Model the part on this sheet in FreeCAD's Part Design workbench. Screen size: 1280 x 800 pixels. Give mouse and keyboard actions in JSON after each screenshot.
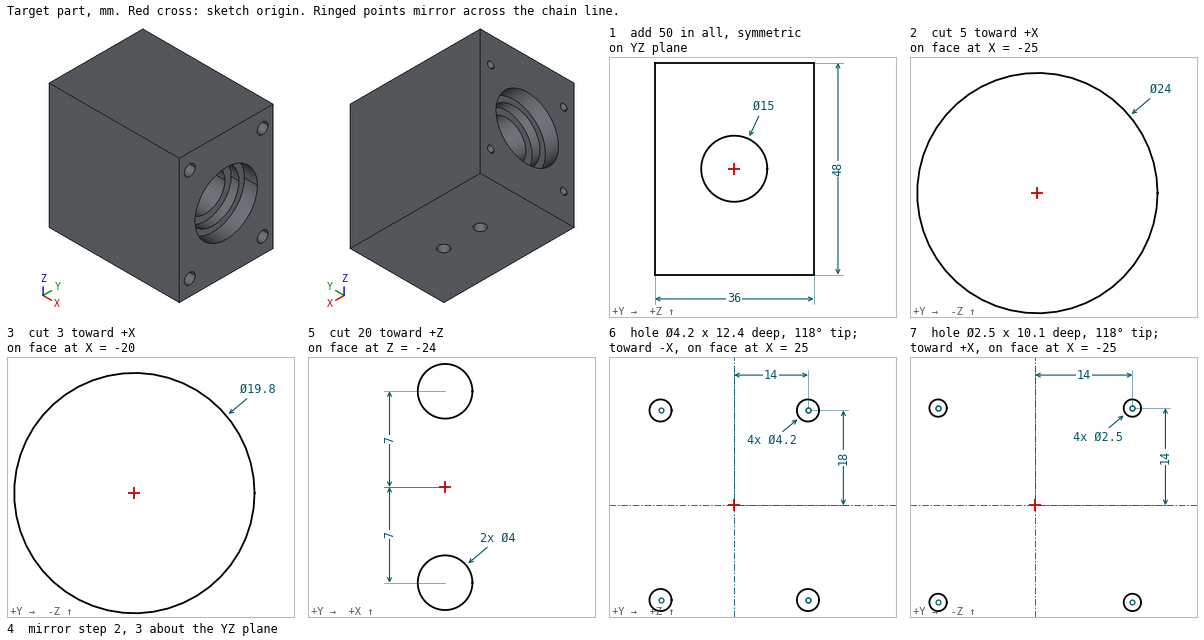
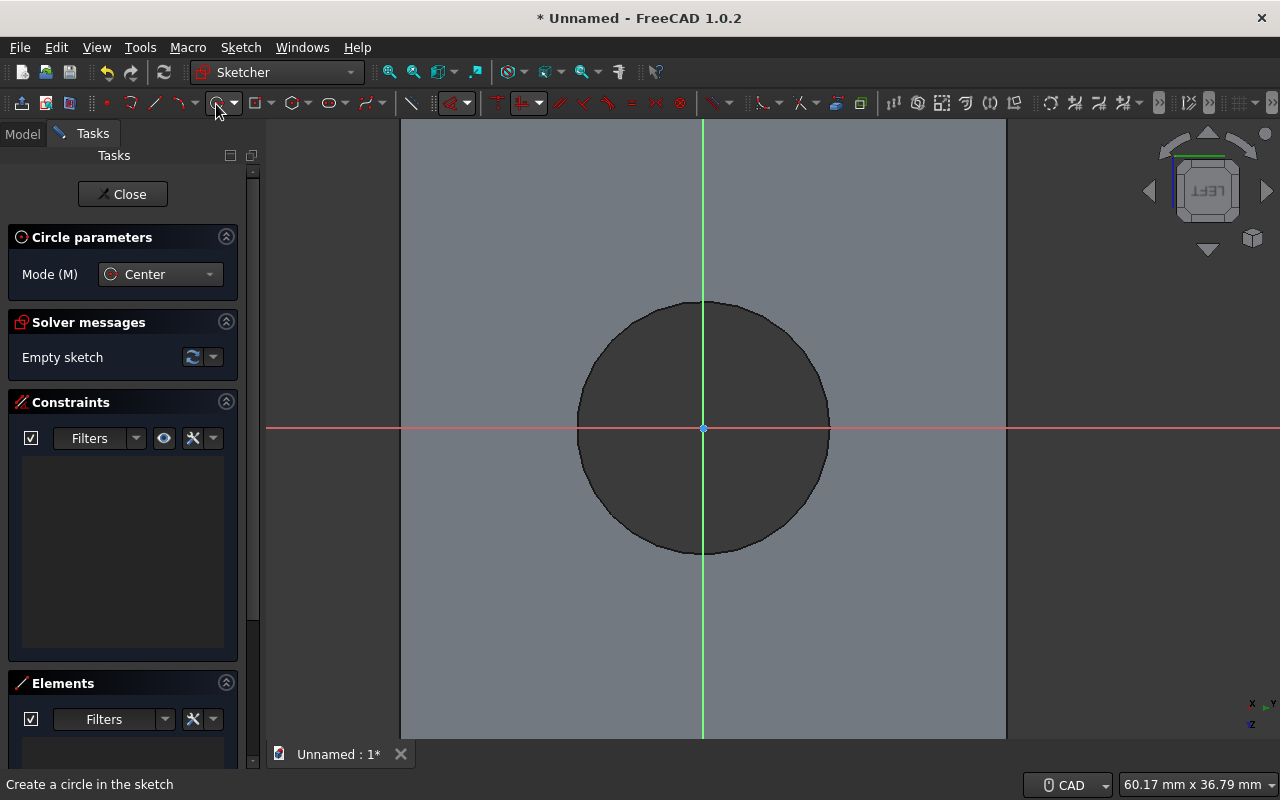
{"action": "left_click", "coordinate": [703, 428]}
{"action": "left_click", "coordinate": [846, 285]}
{"action": "key", "text": "Escape"}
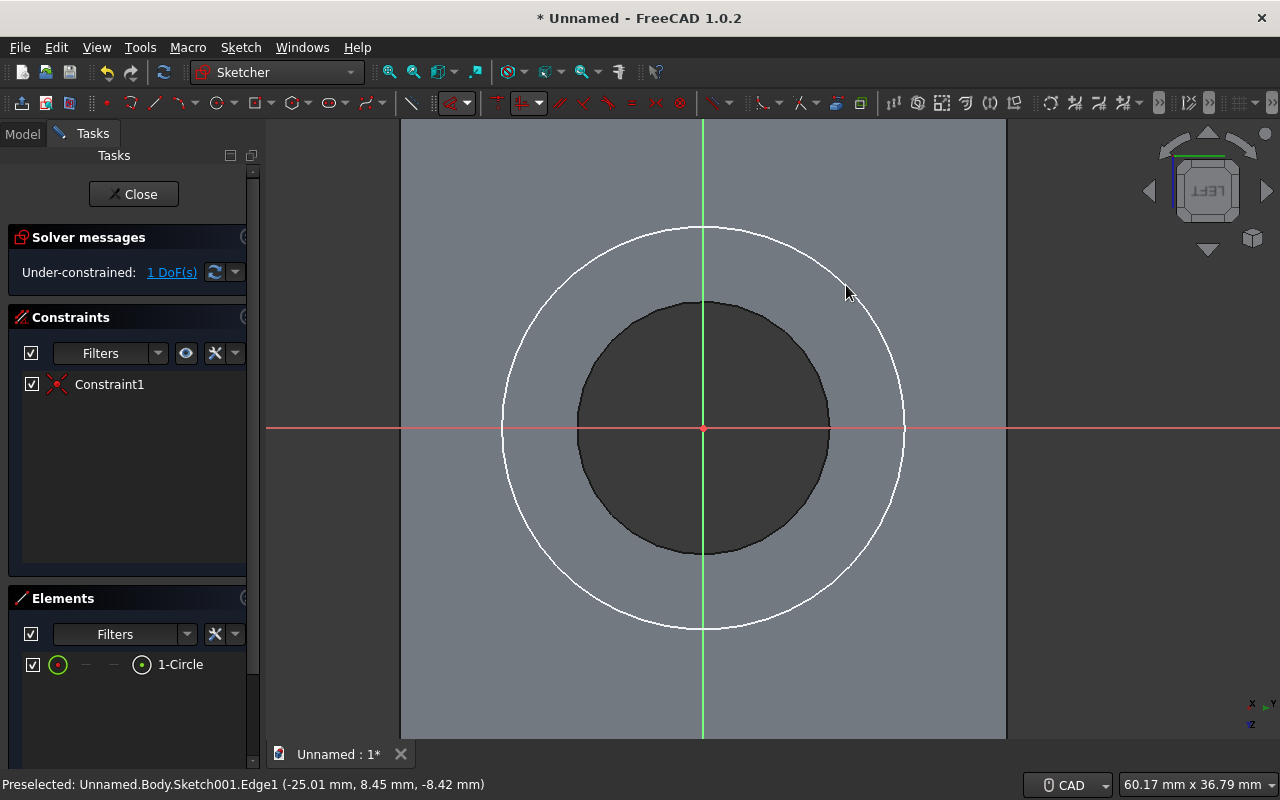
{"action": "left_click", "coordinate": [845, 285]}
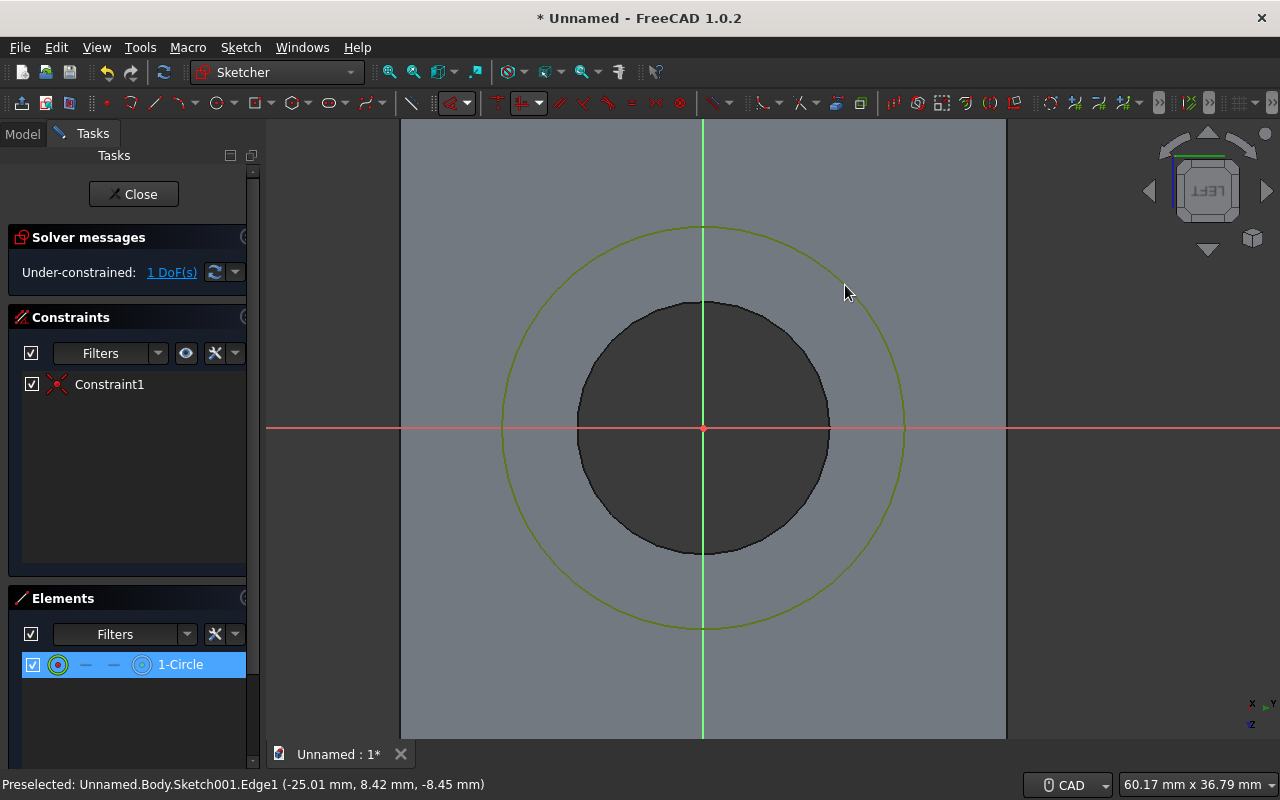
{"action": "key", "text": "k o"}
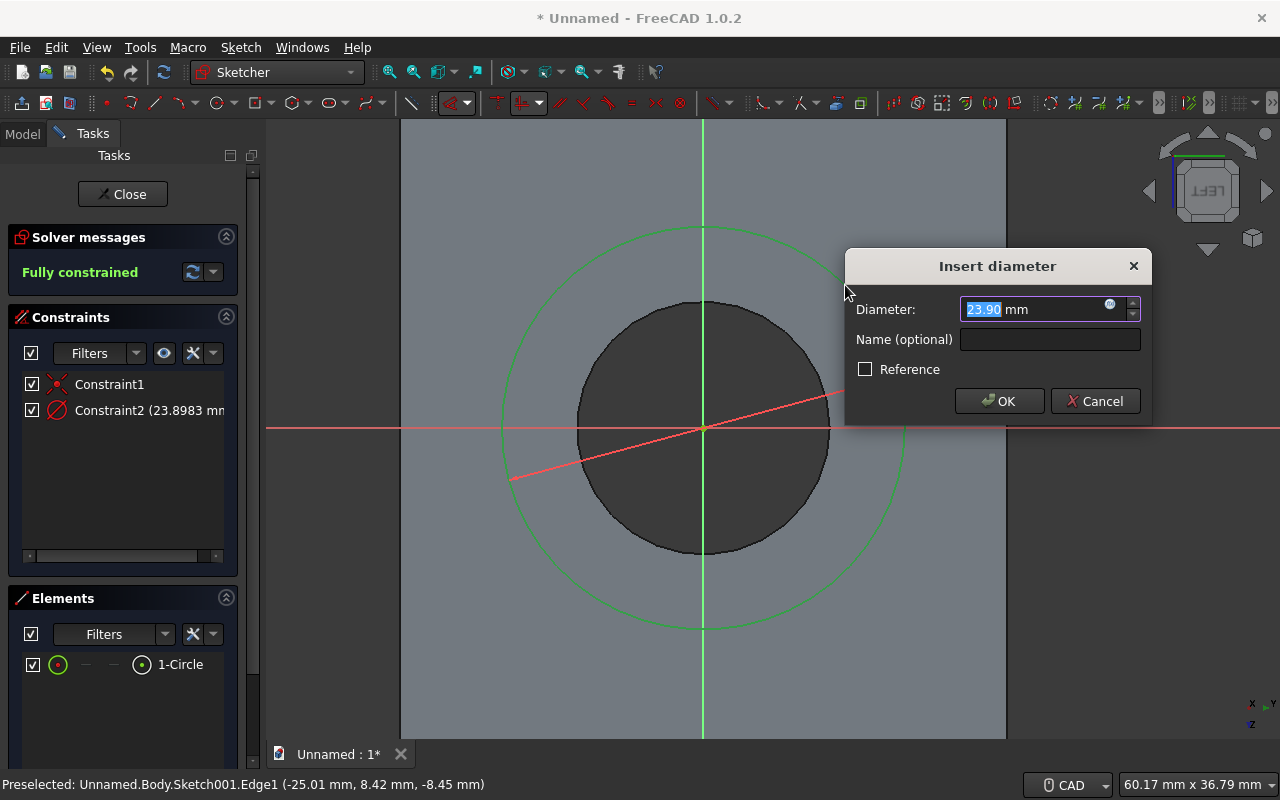
{"action": "type", "text": "24"}
{"action": "key", "text": "Return"}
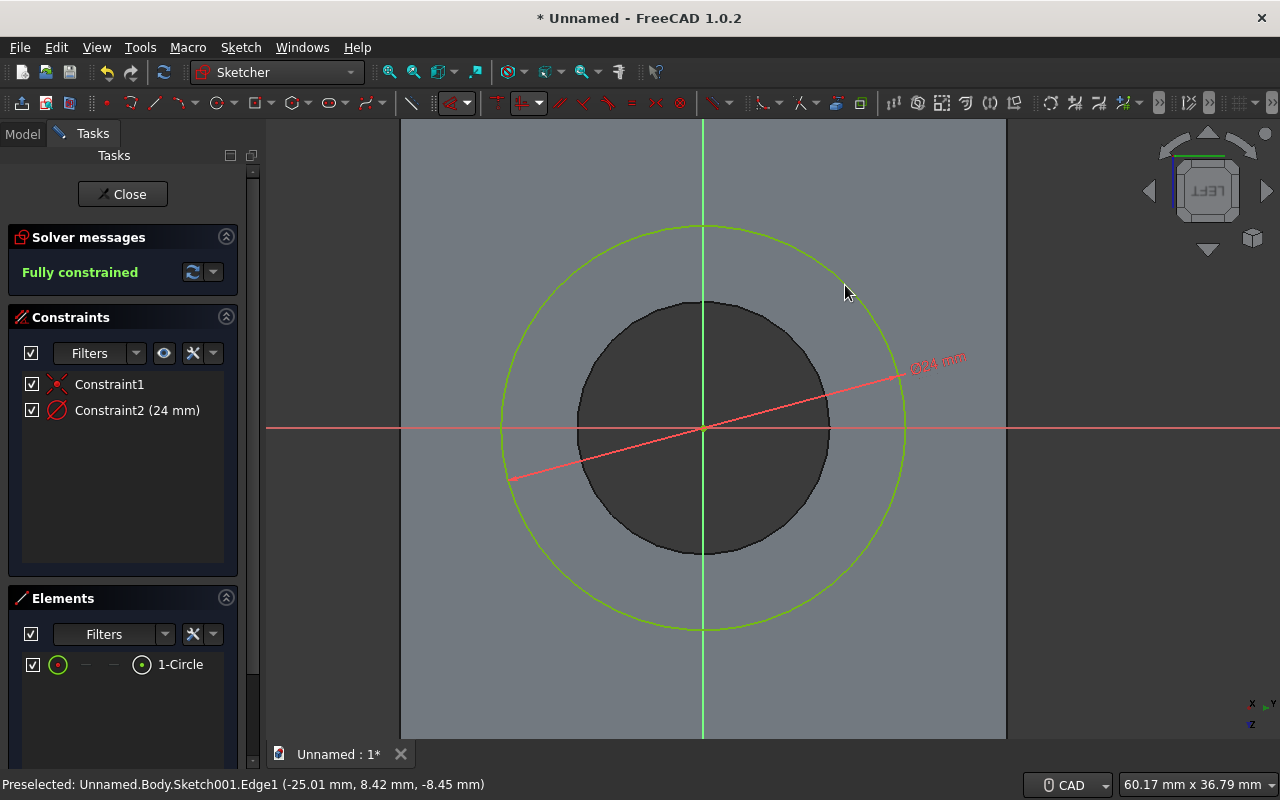
{"action": "left_click", "coordinate": [123, 194]}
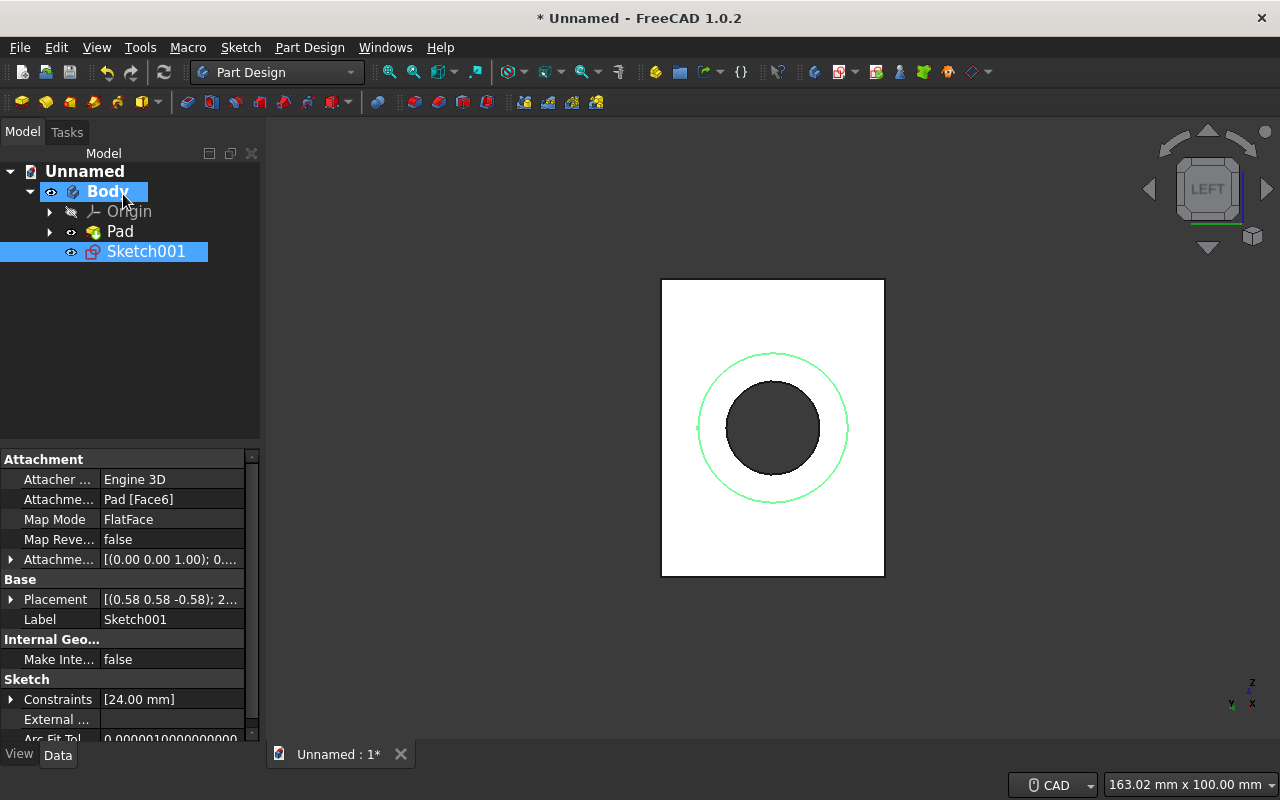
{"action": "left_click", "coordinate": [188, 102]}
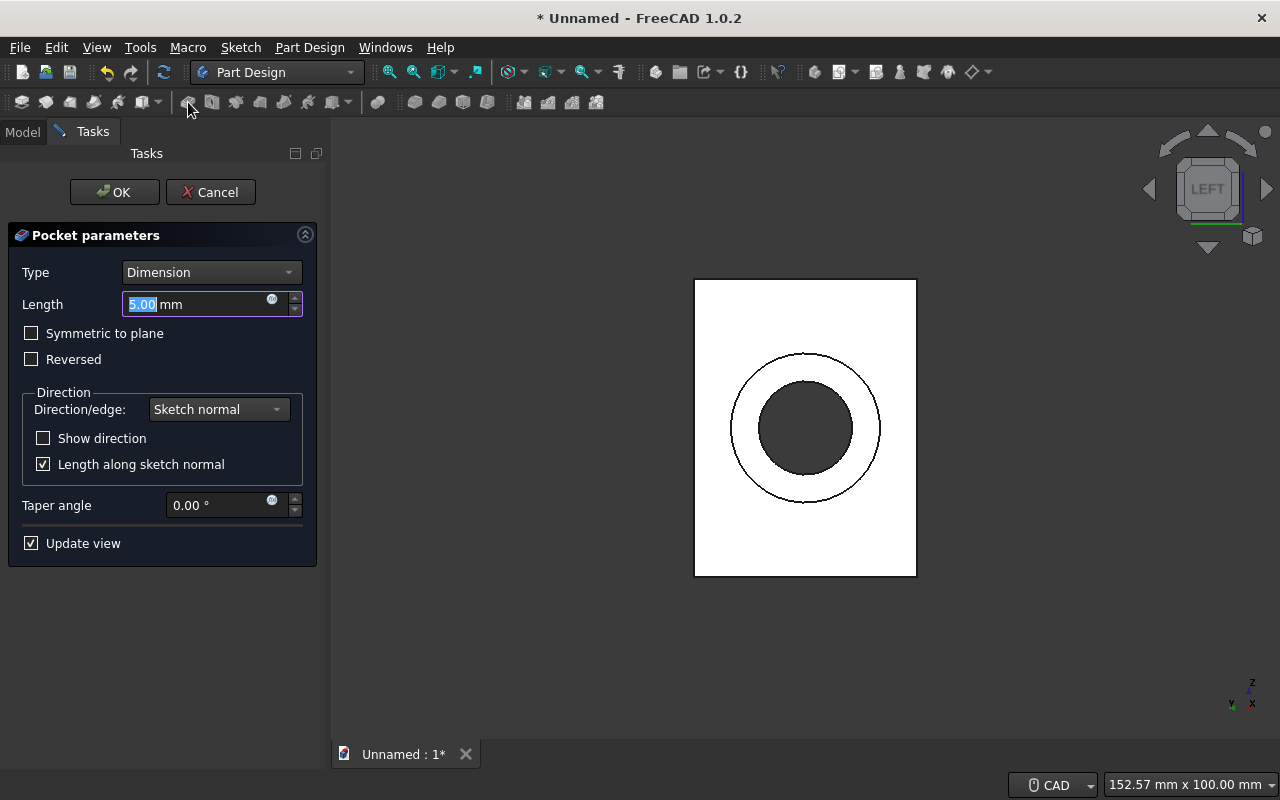
{"action": "type", "text": "5"}
{"action": "key", "text": "Tab"}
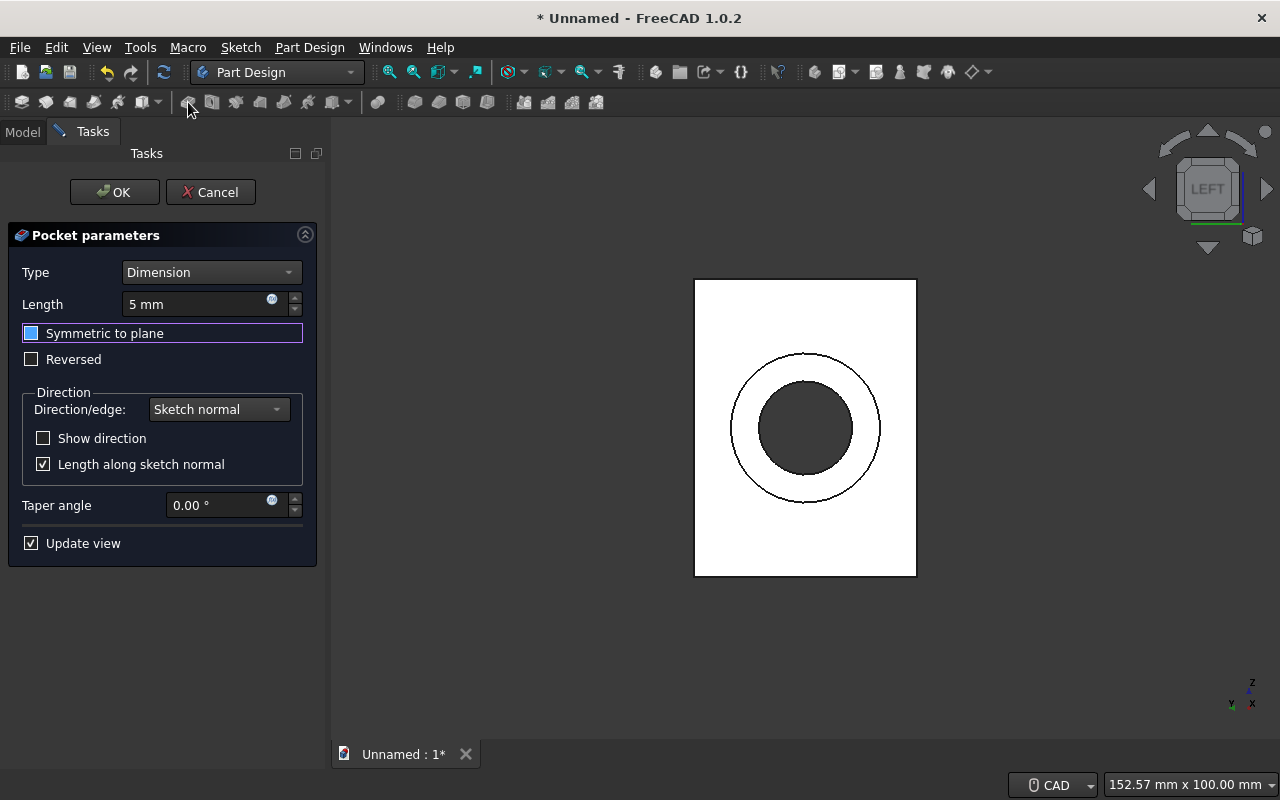
{"action": "left_click", "coordinate": [115, 192]}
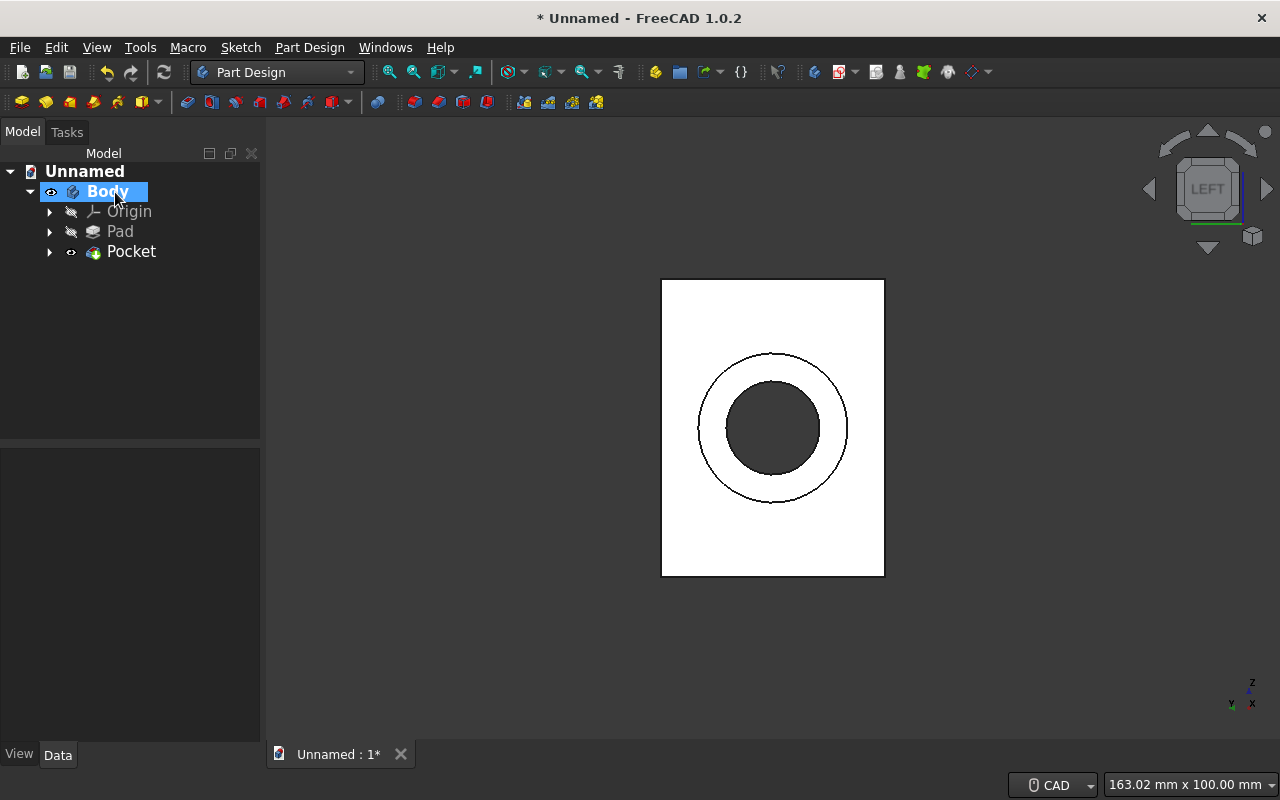
{"action": "left_click", "coordinate": [730, 470]}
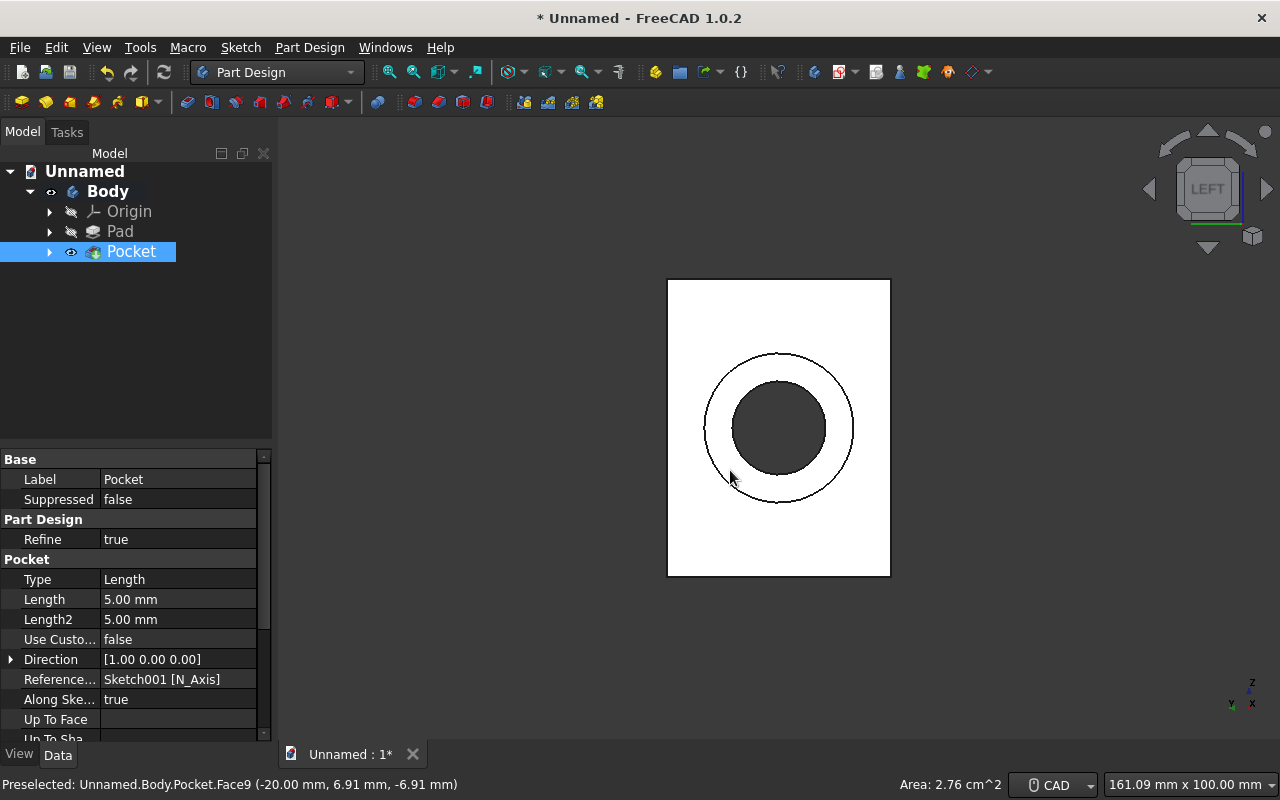
{"action": "left_click", "coordinate": [840, 72]}